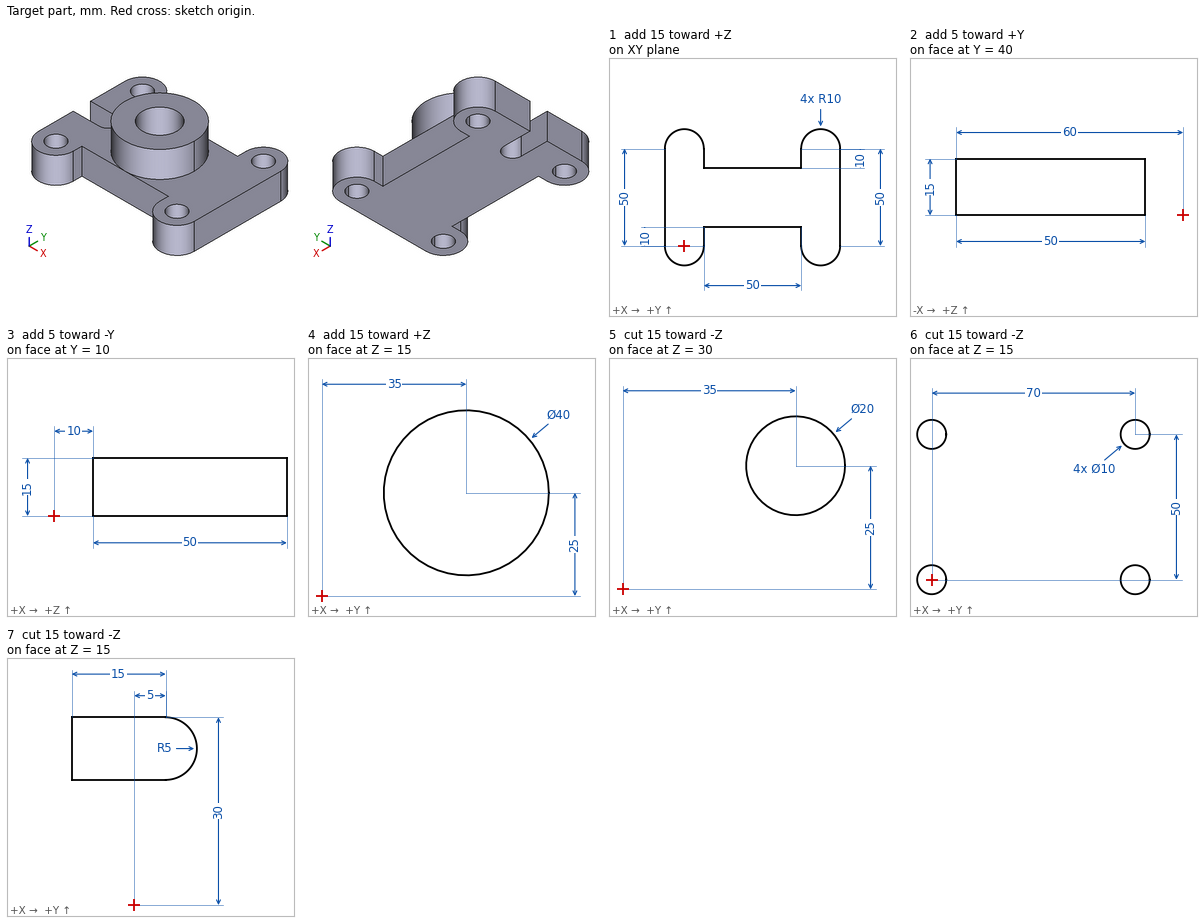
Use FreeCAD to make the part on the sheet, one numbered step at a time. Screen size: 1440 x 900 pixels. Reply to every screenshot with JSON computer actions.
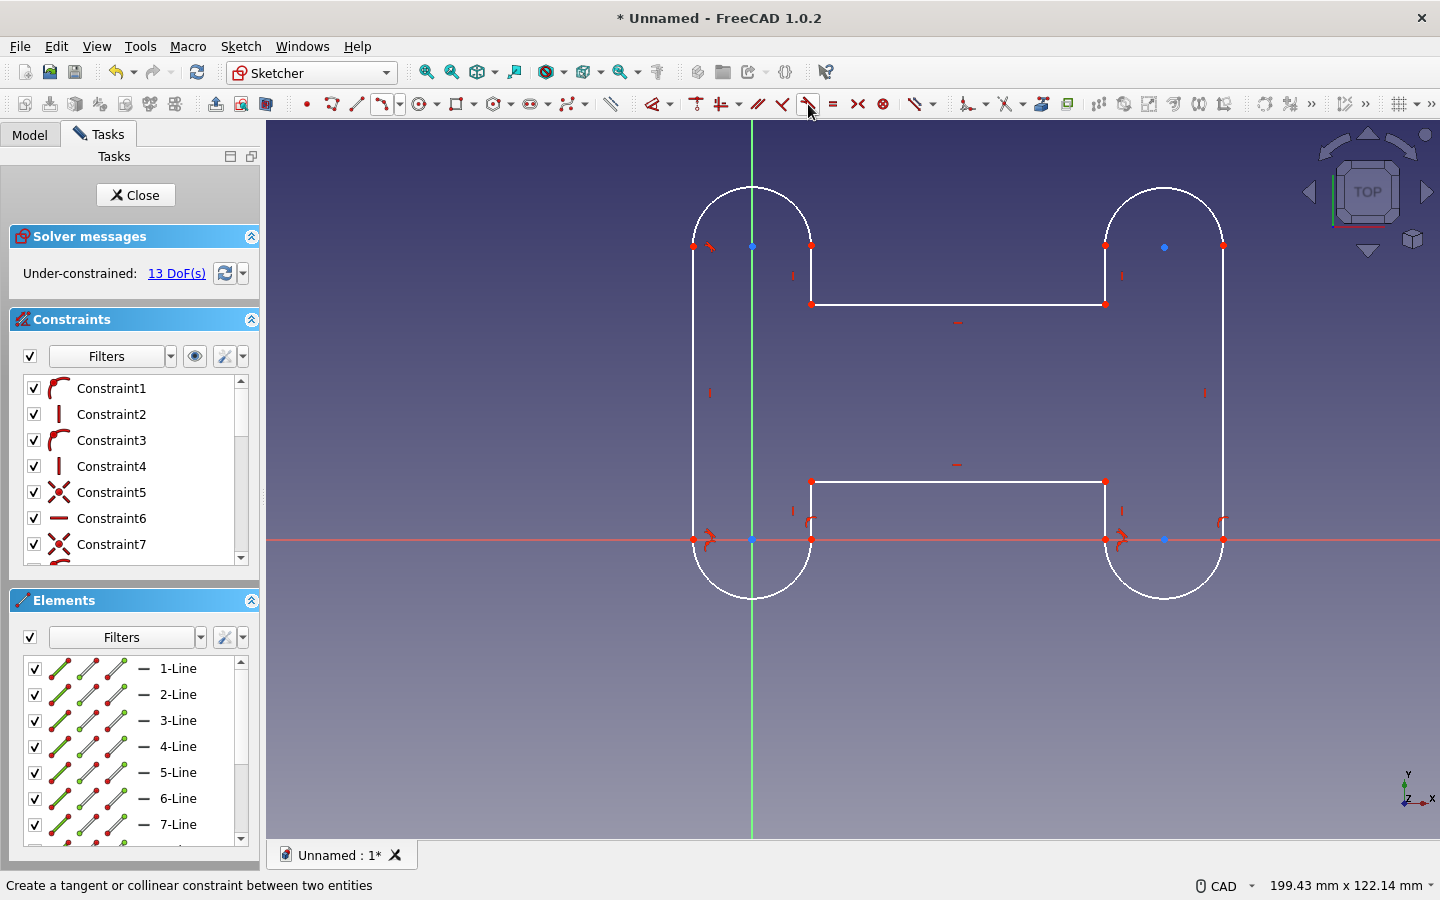
{"action": "left_click", "coordinate": [1223, 452]}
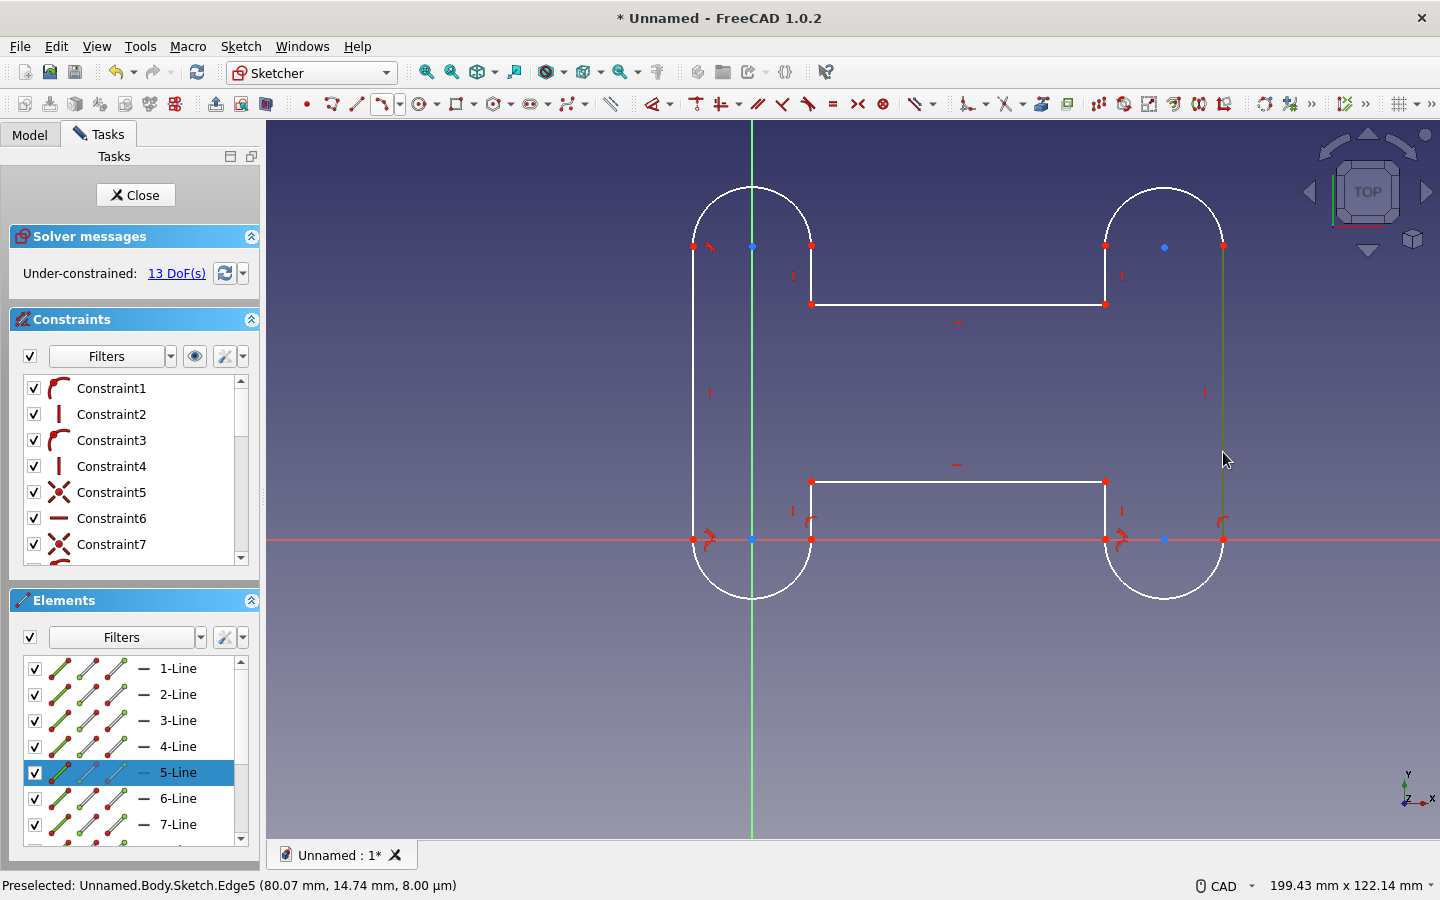
{"action": "left_click", "coordinate": [1198, 199]}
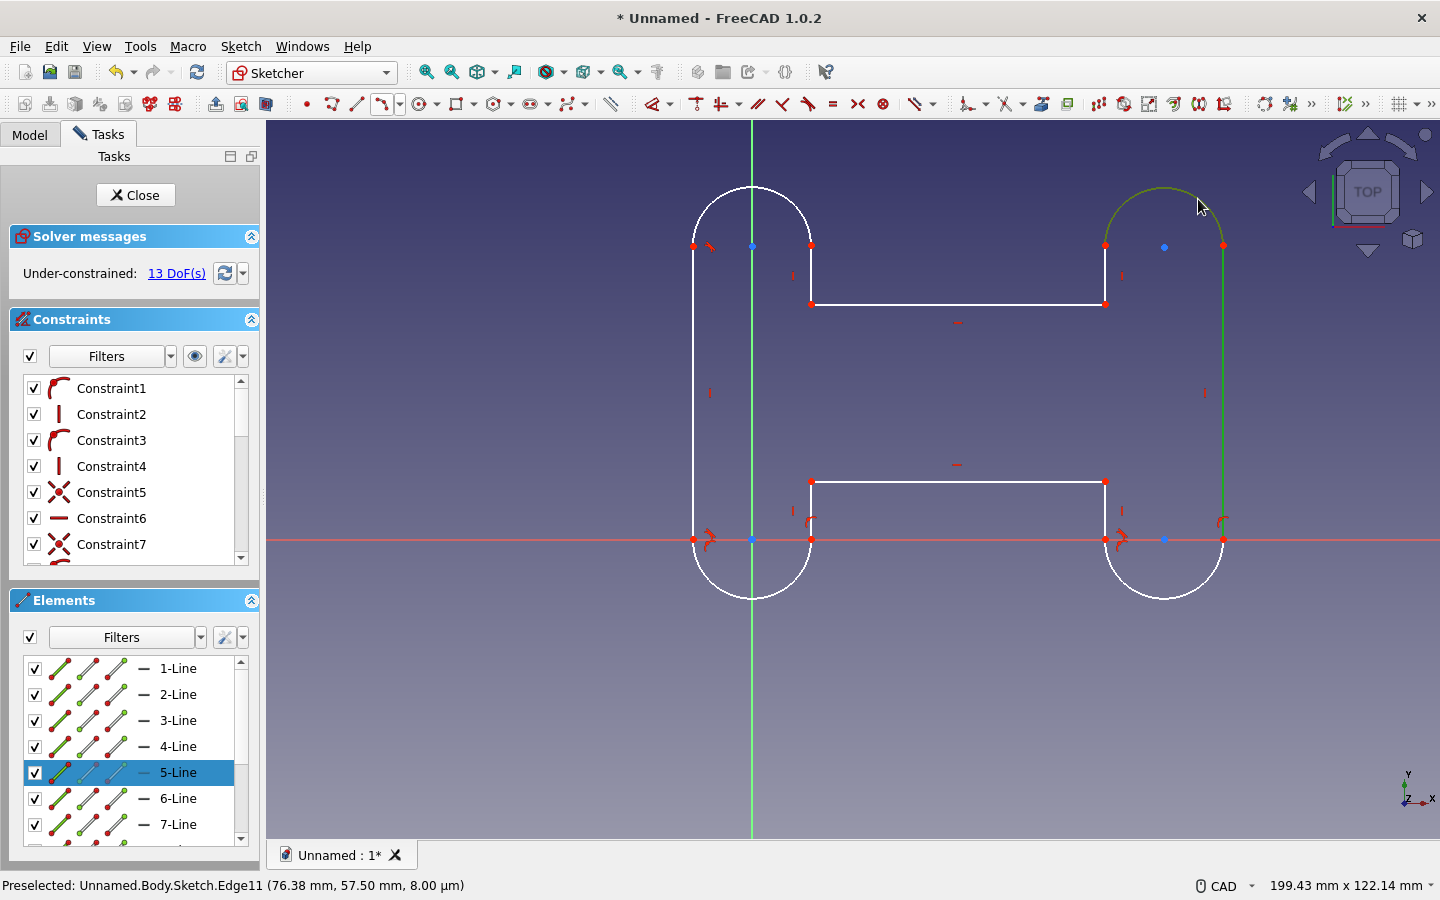
{"action": "key", "text": "t"}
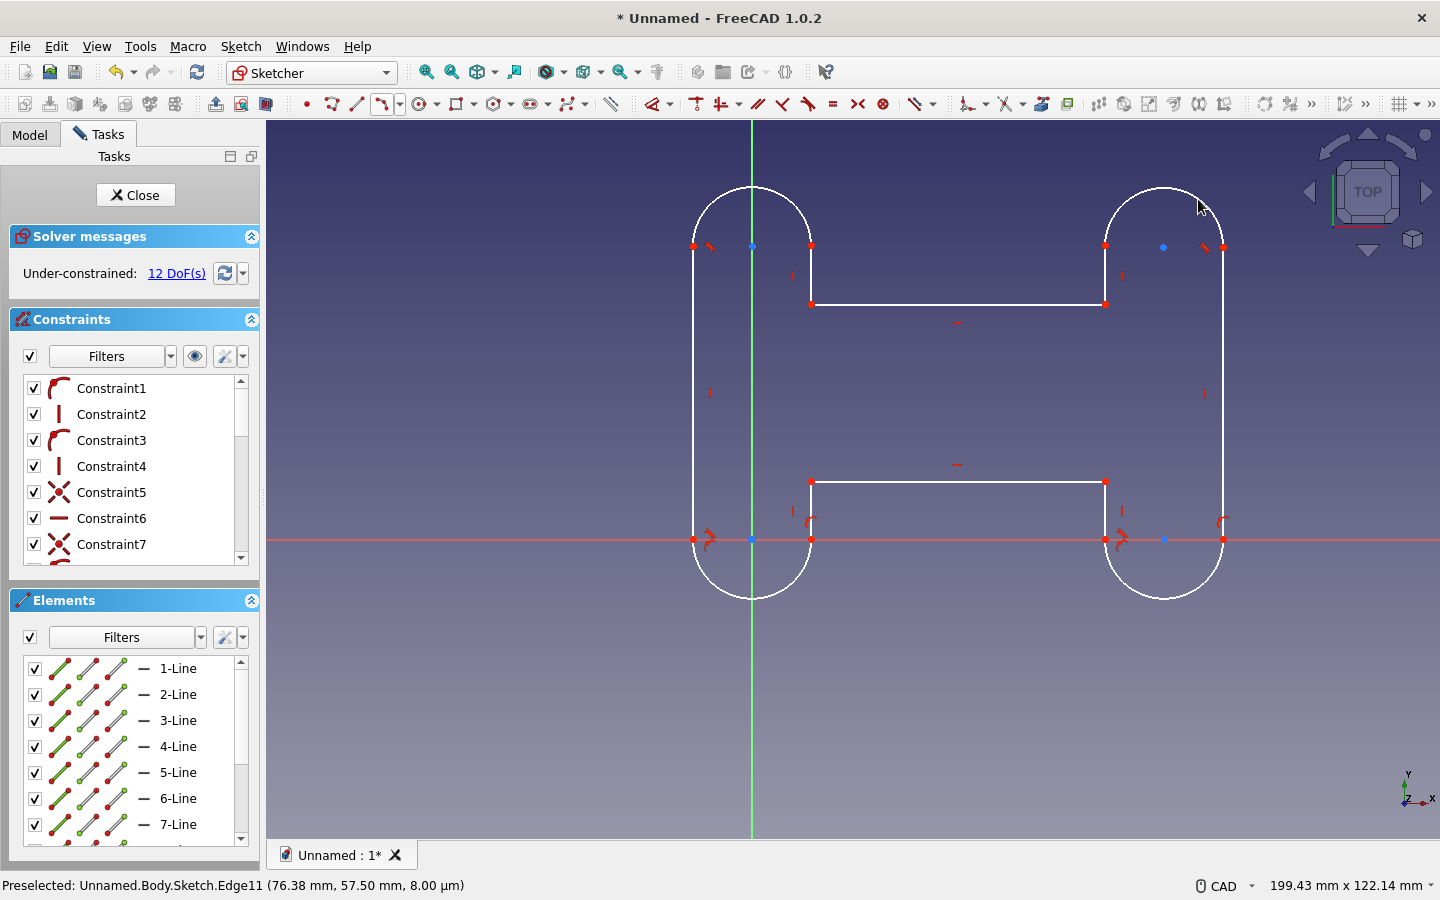
{"action": "left_click", "coordinate": [1105, 264]}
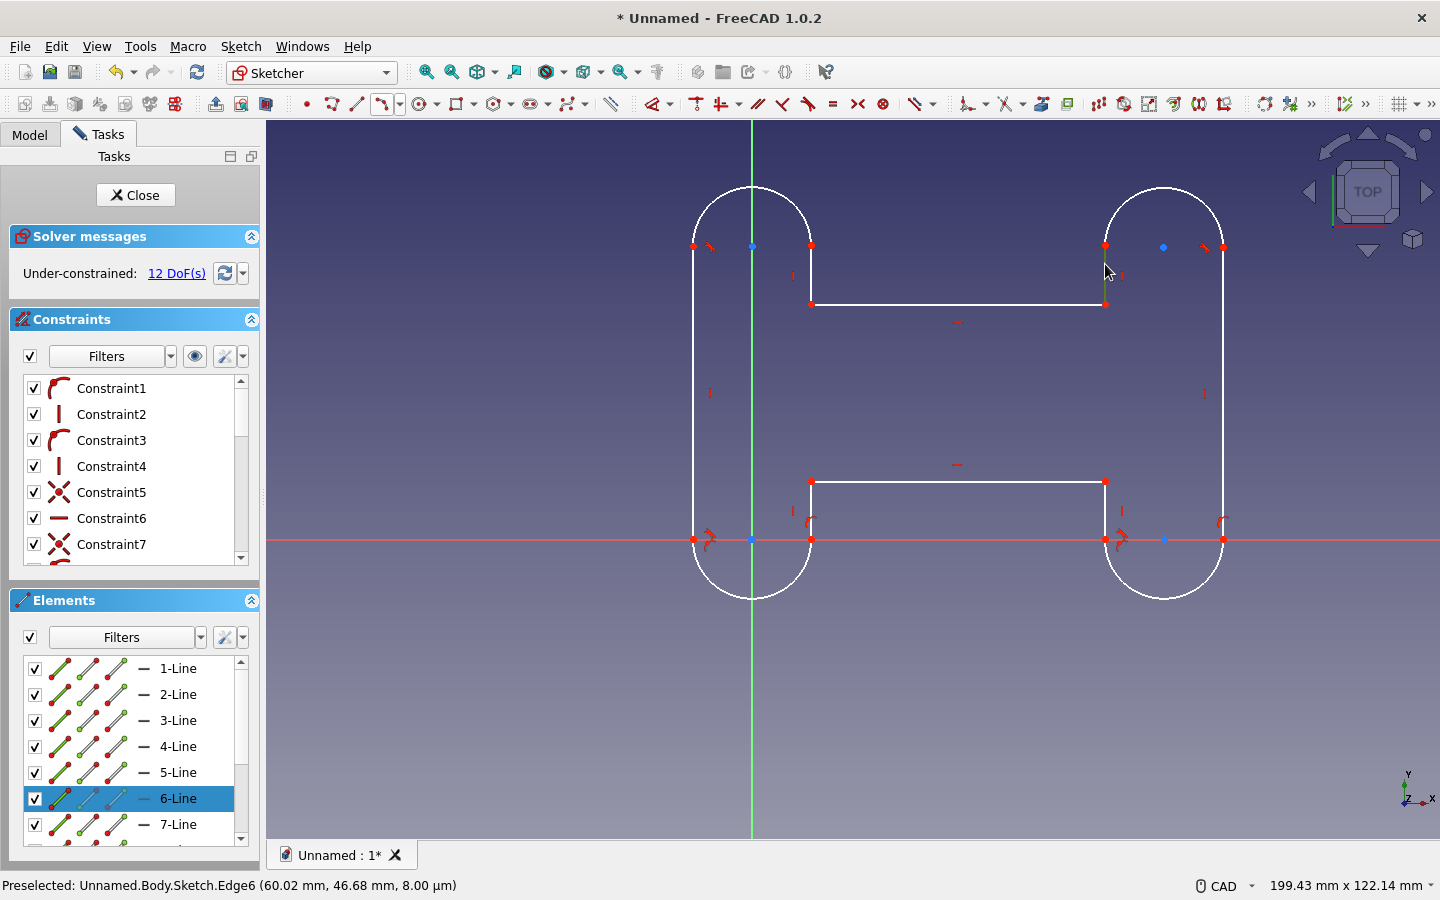
{"action": "left_click", "coordinate": [1199, 199]}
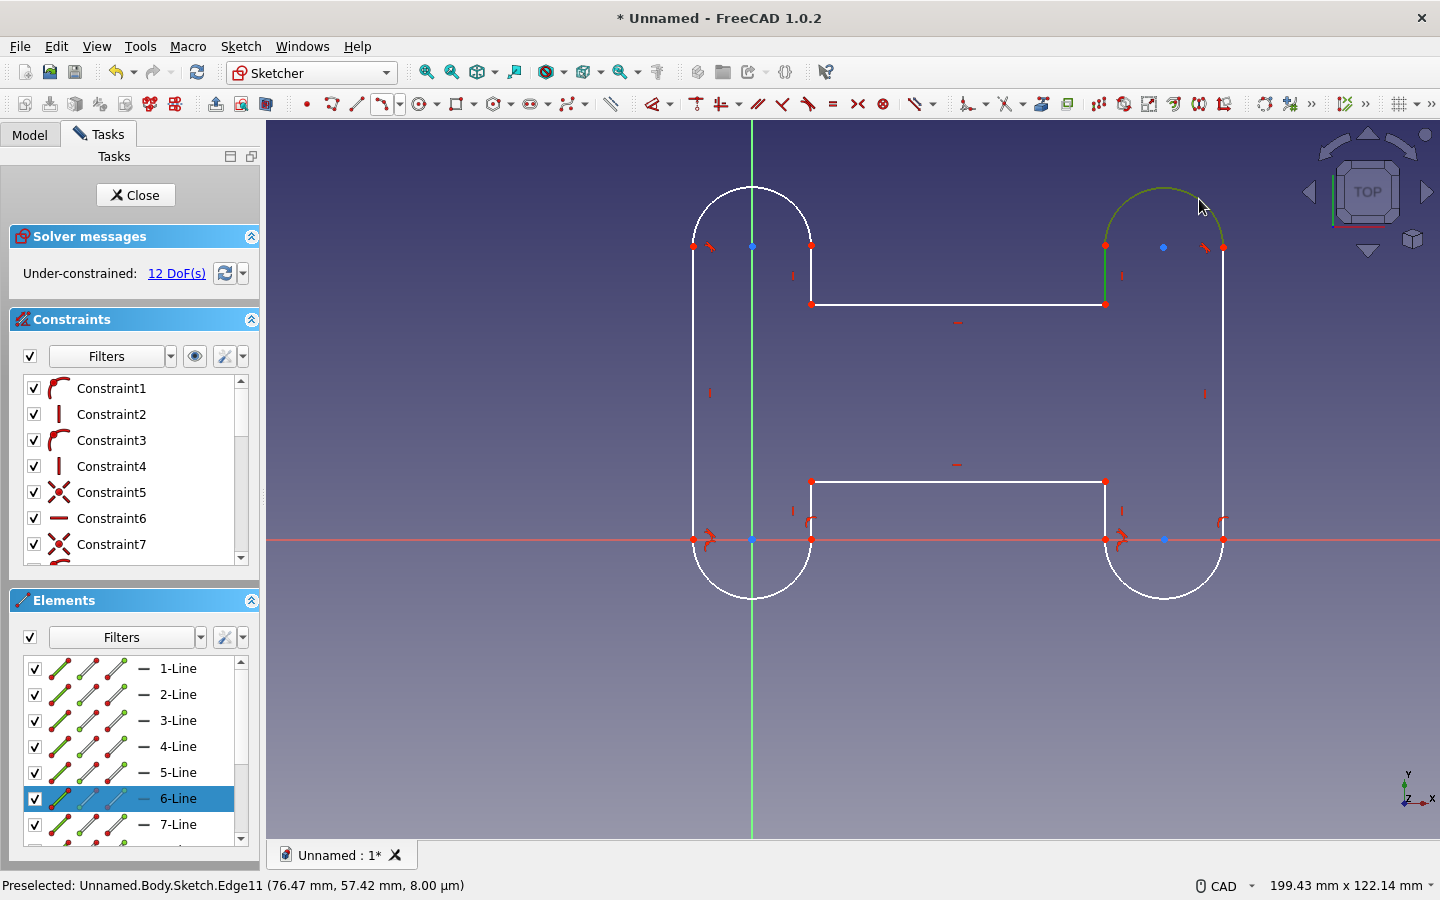
{"action": "key", "text": "t"}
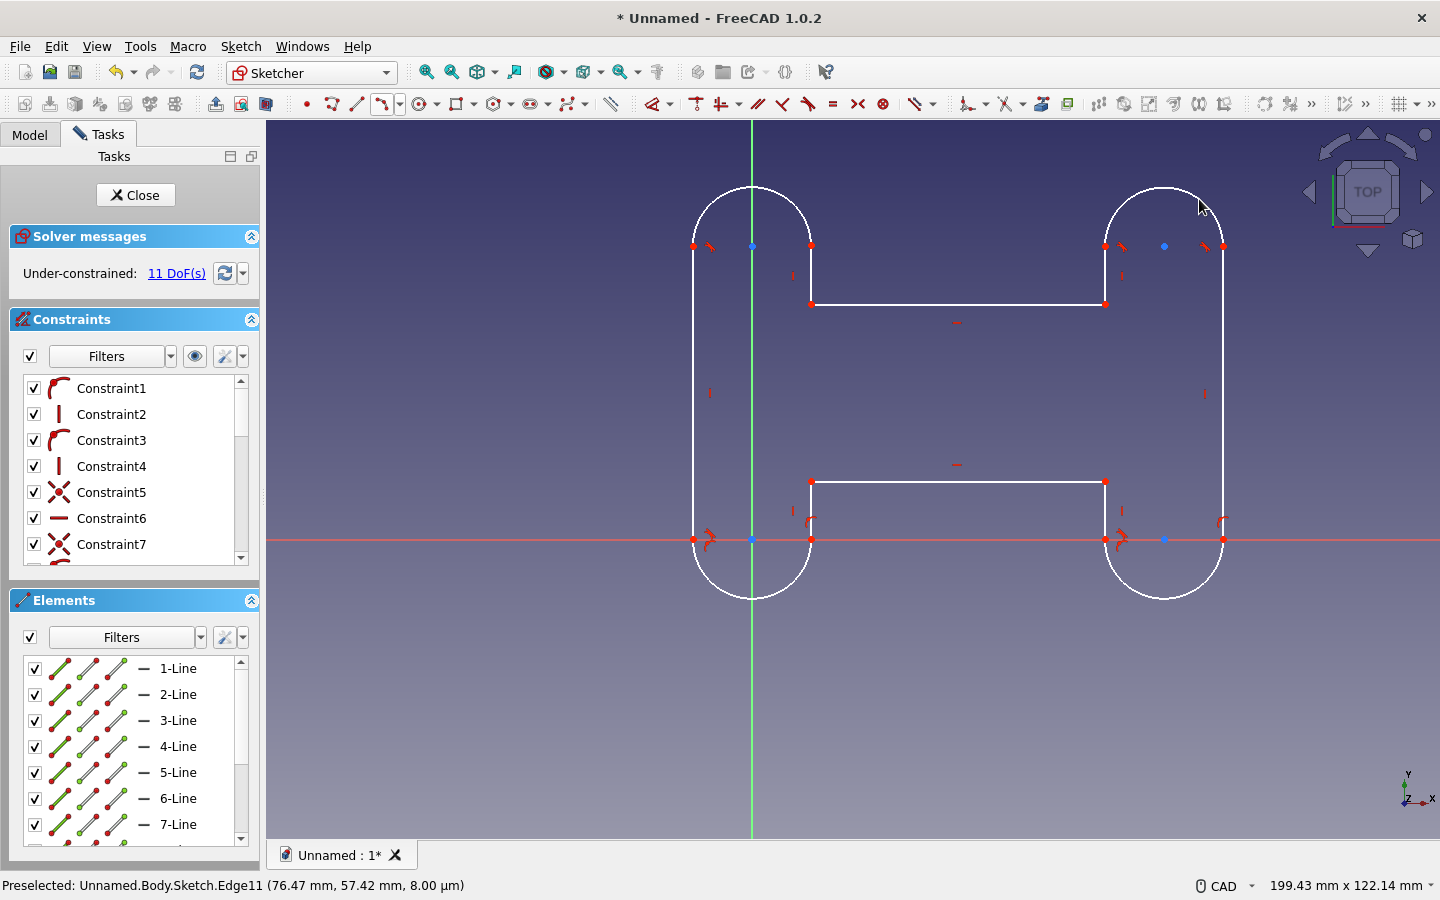
{"action": "left_click", "coordinate": [811, 287]}